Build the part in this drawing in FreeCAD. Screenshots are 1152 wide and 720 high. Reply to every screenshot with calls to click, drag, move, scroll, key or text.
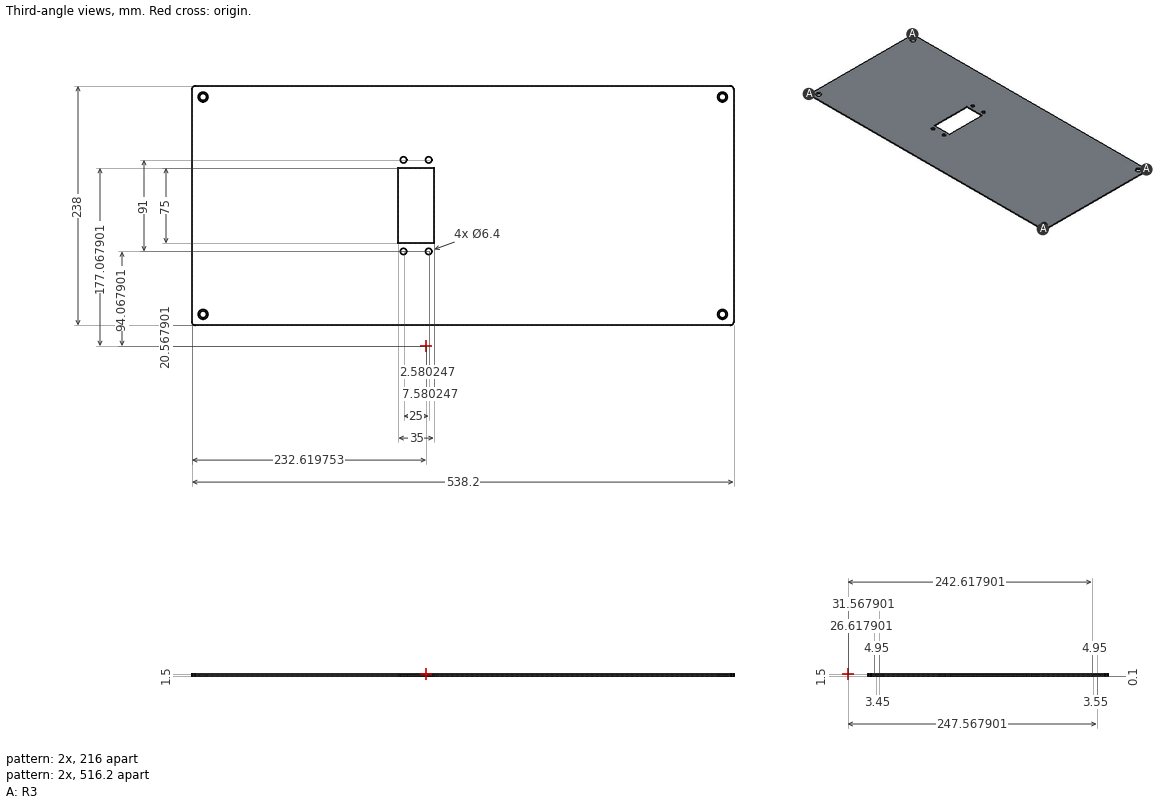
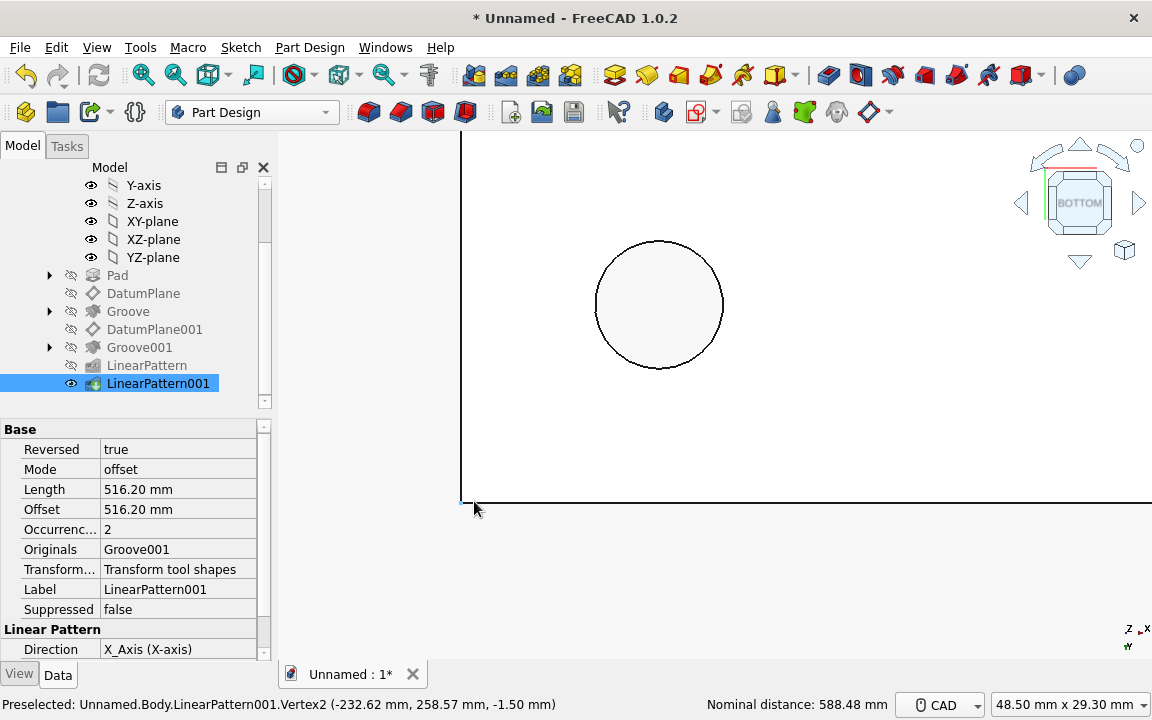
click(144, 76)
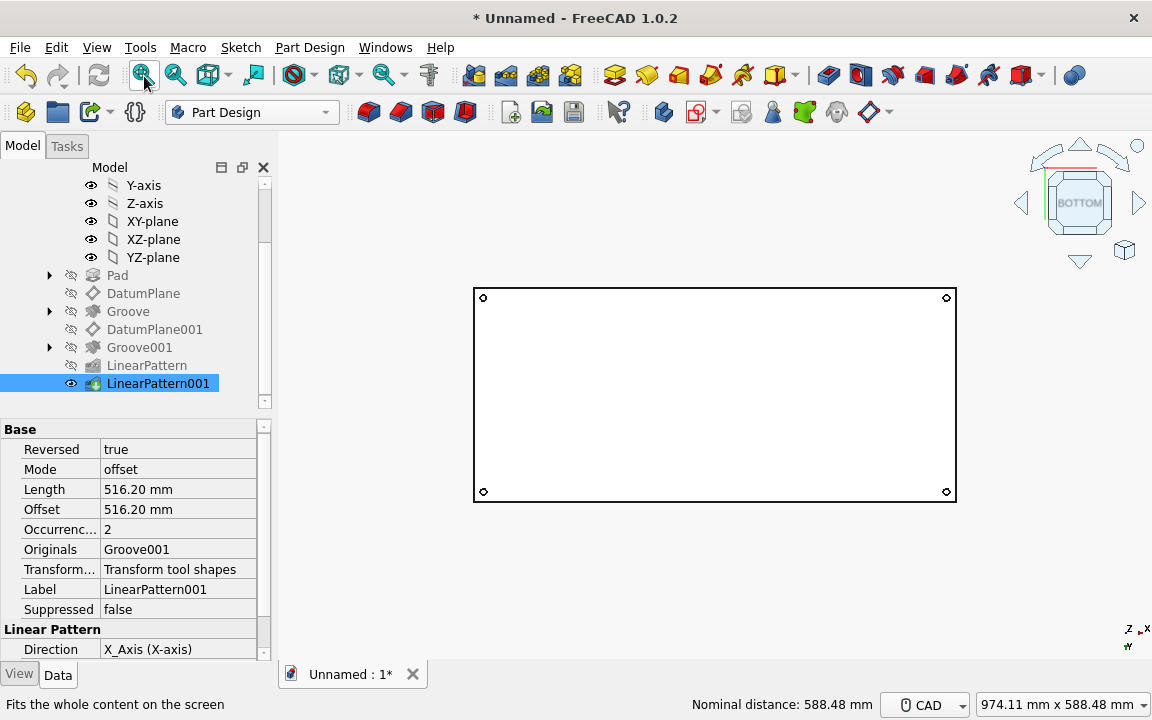
key(4)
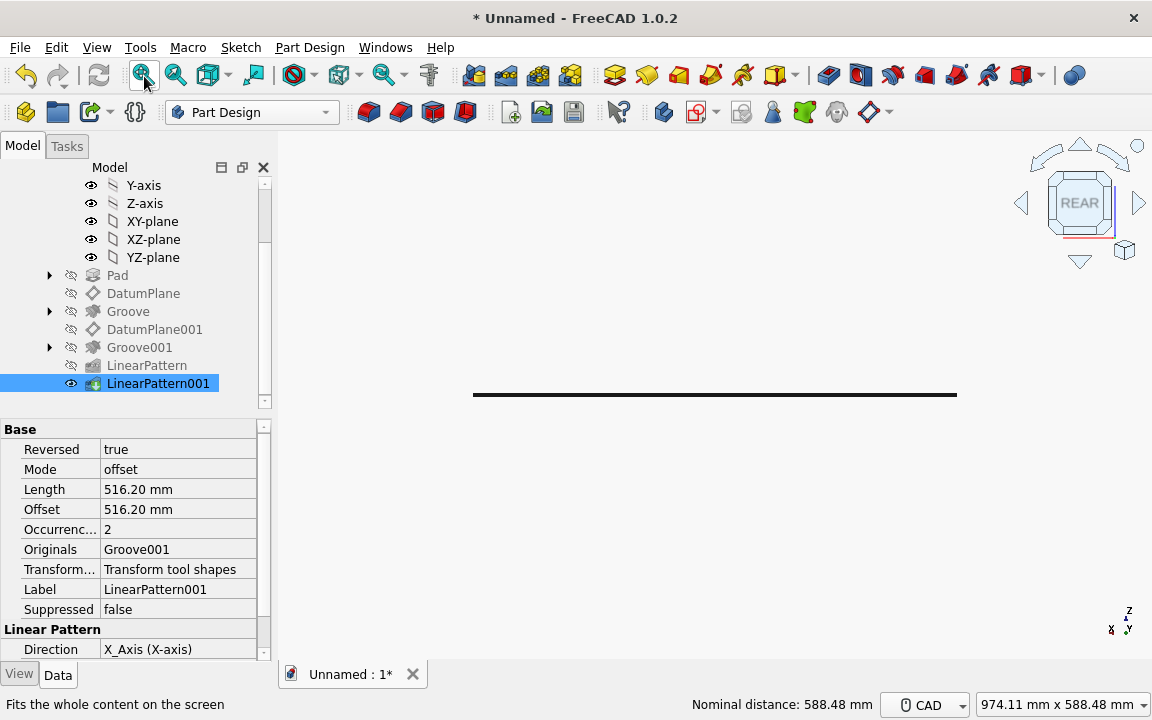
scroll(956, 394, up, 15)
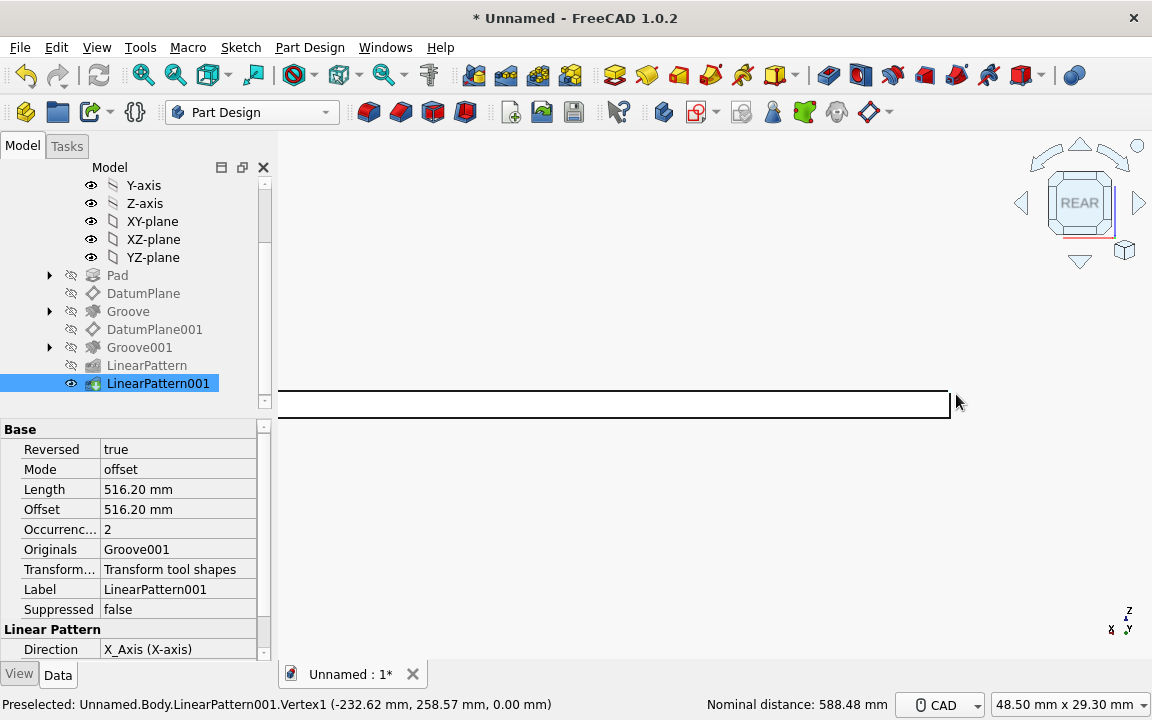
click(950, 404, ctrl)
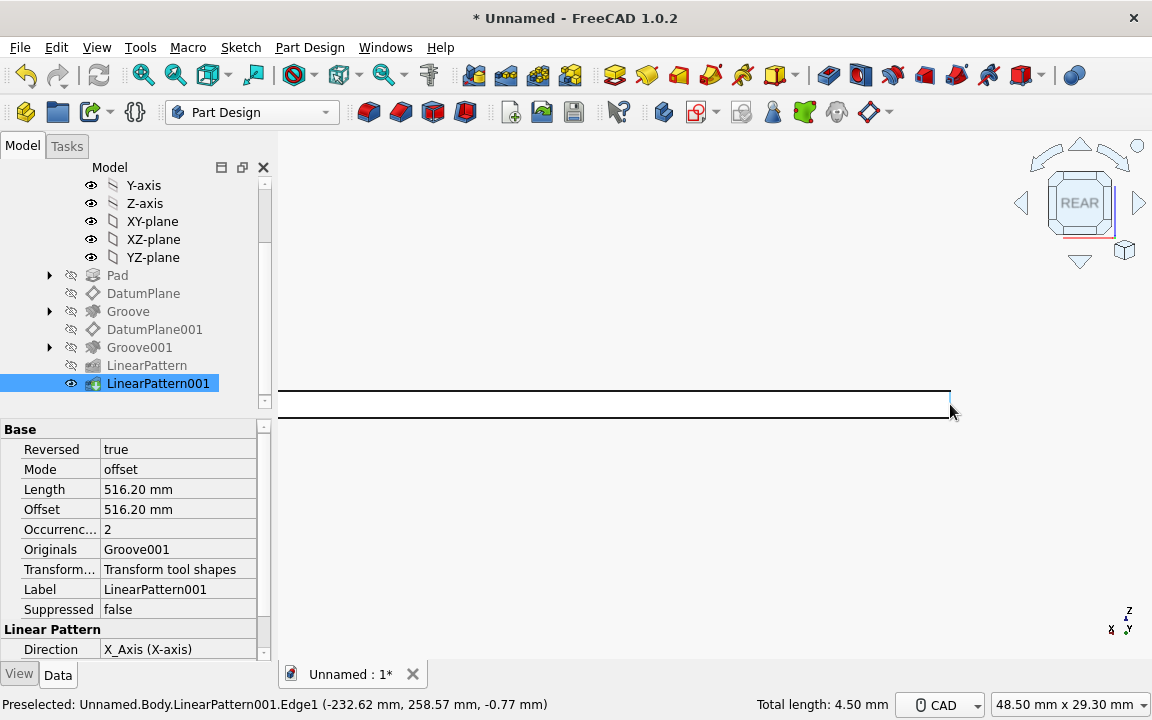
click(144, 76)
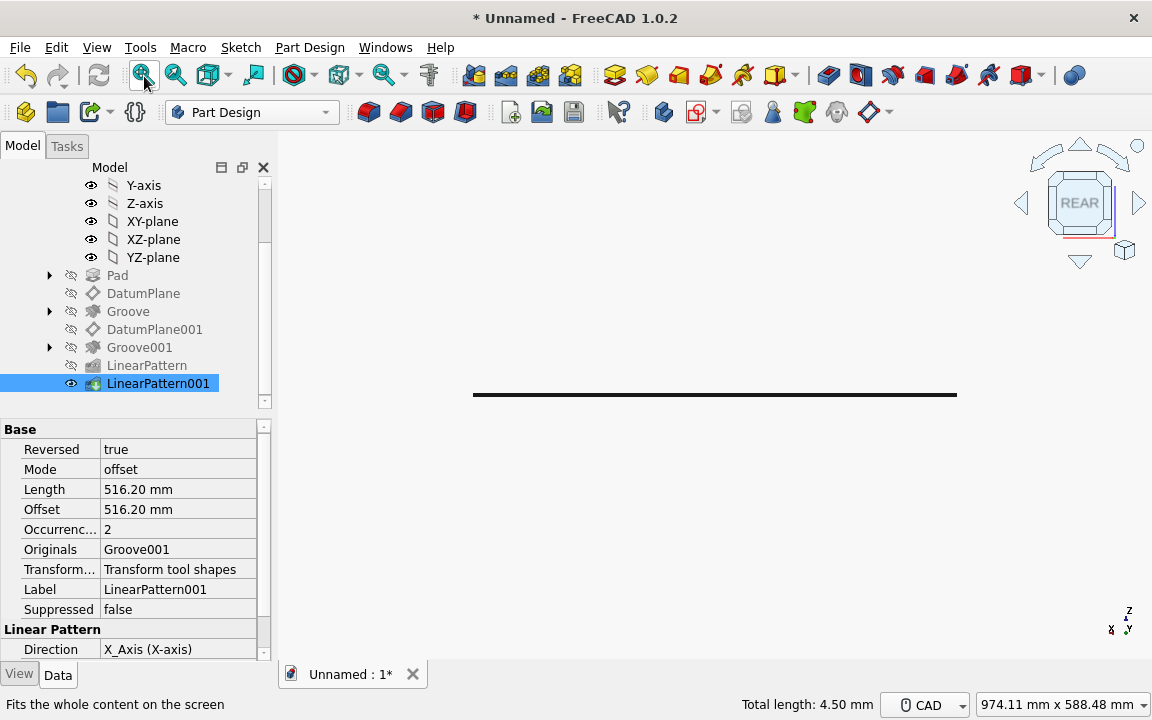
key(6)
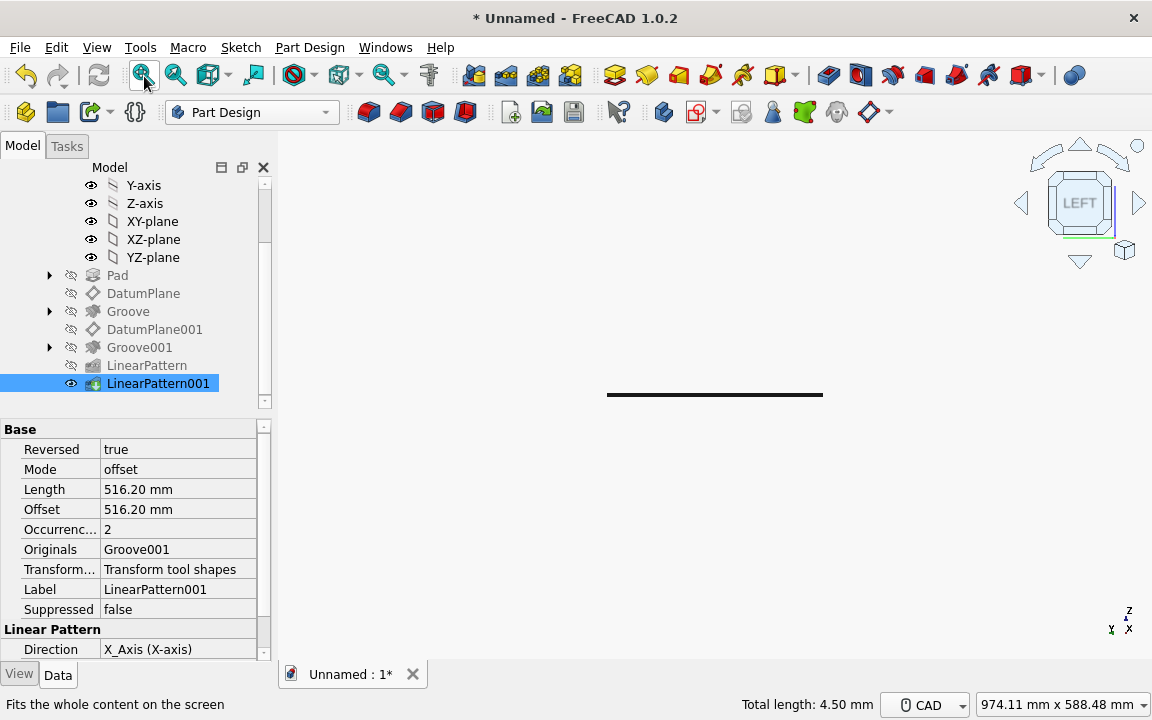
click(144, 76)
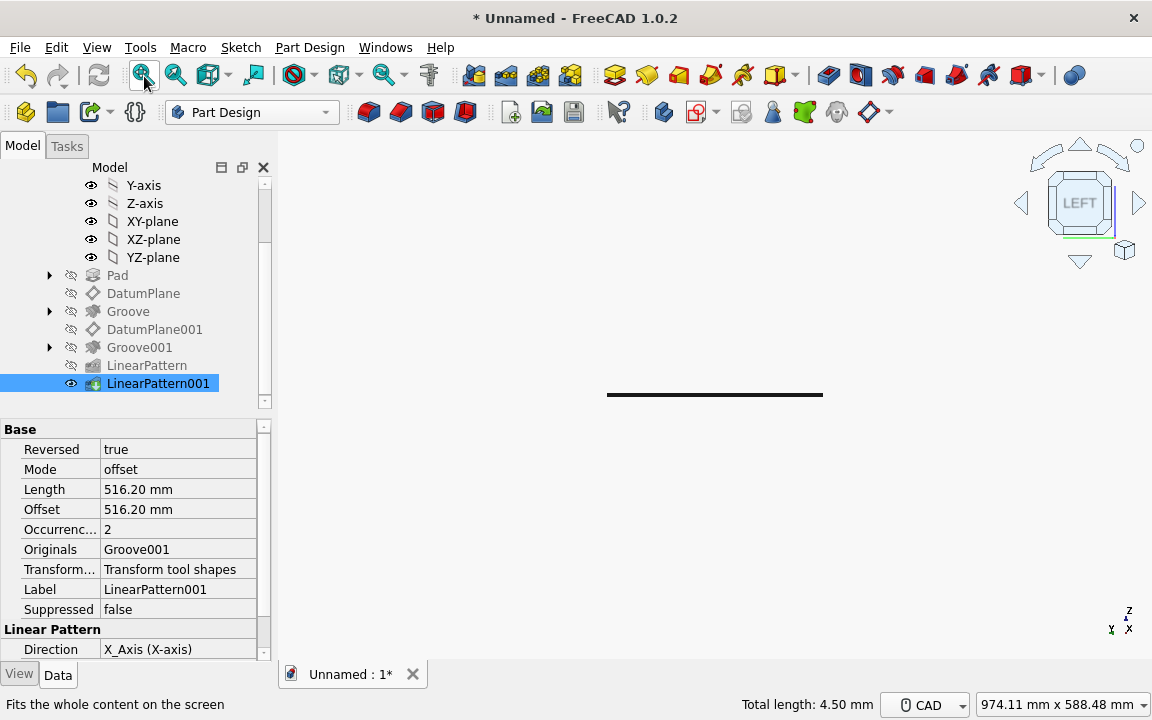
scroll(822, 394, up, 15)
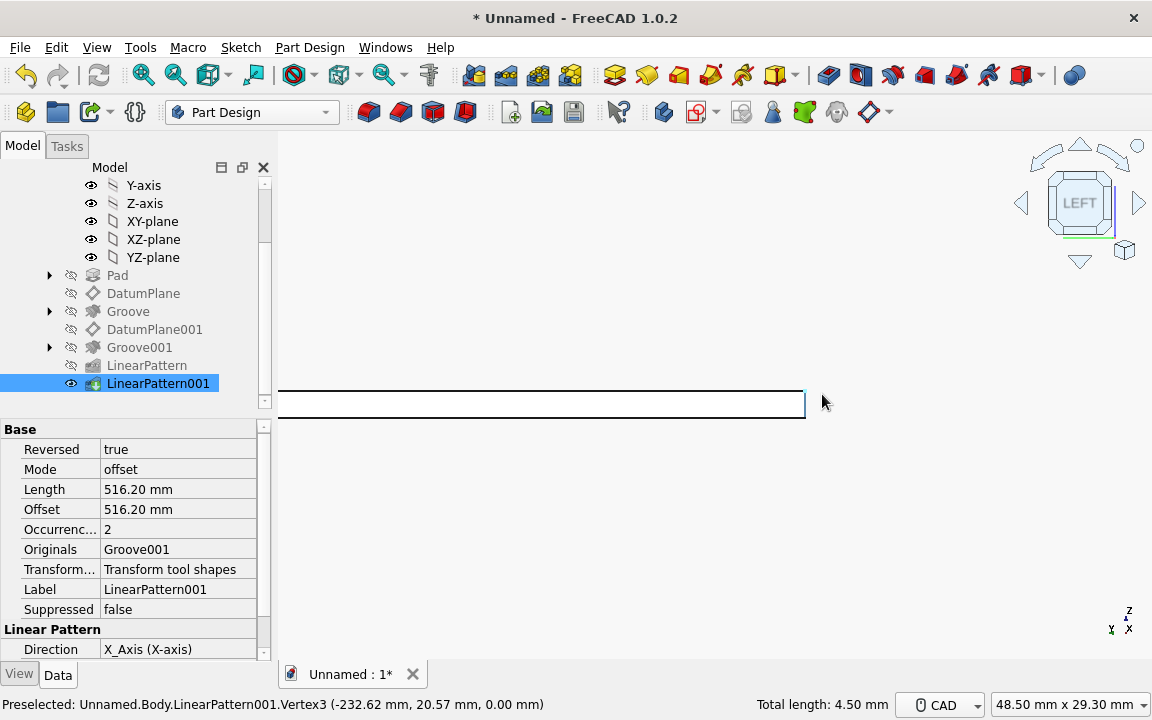
click(144, 76)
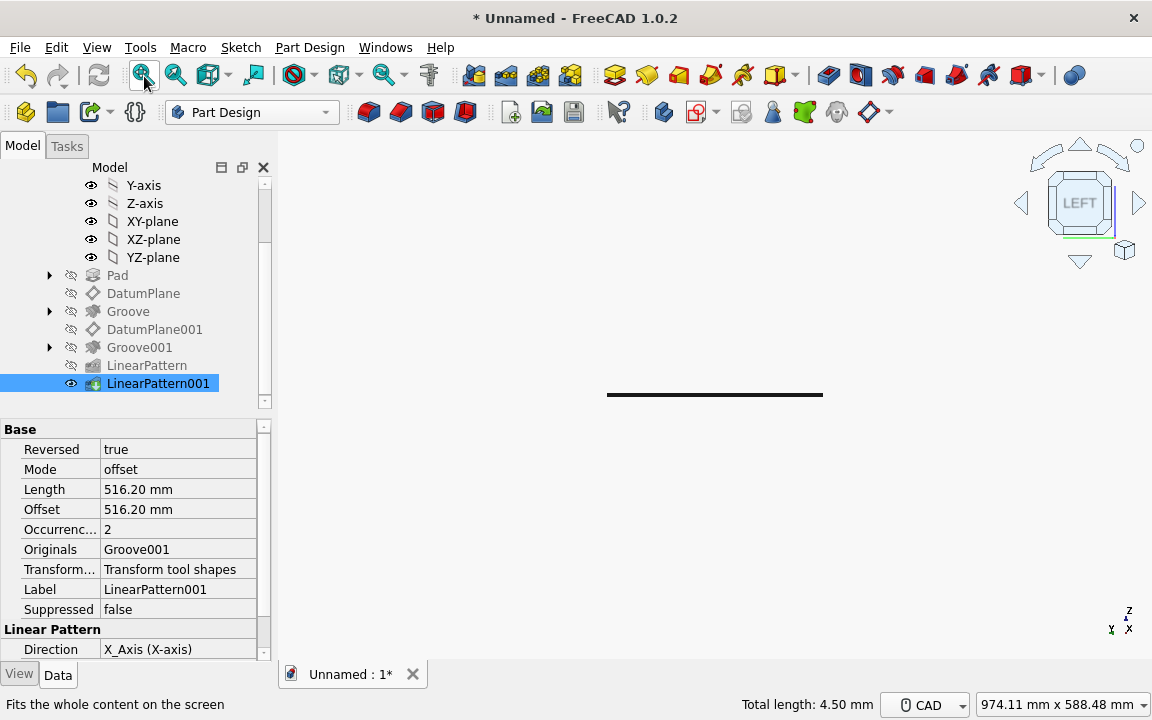
key(v)
key(3)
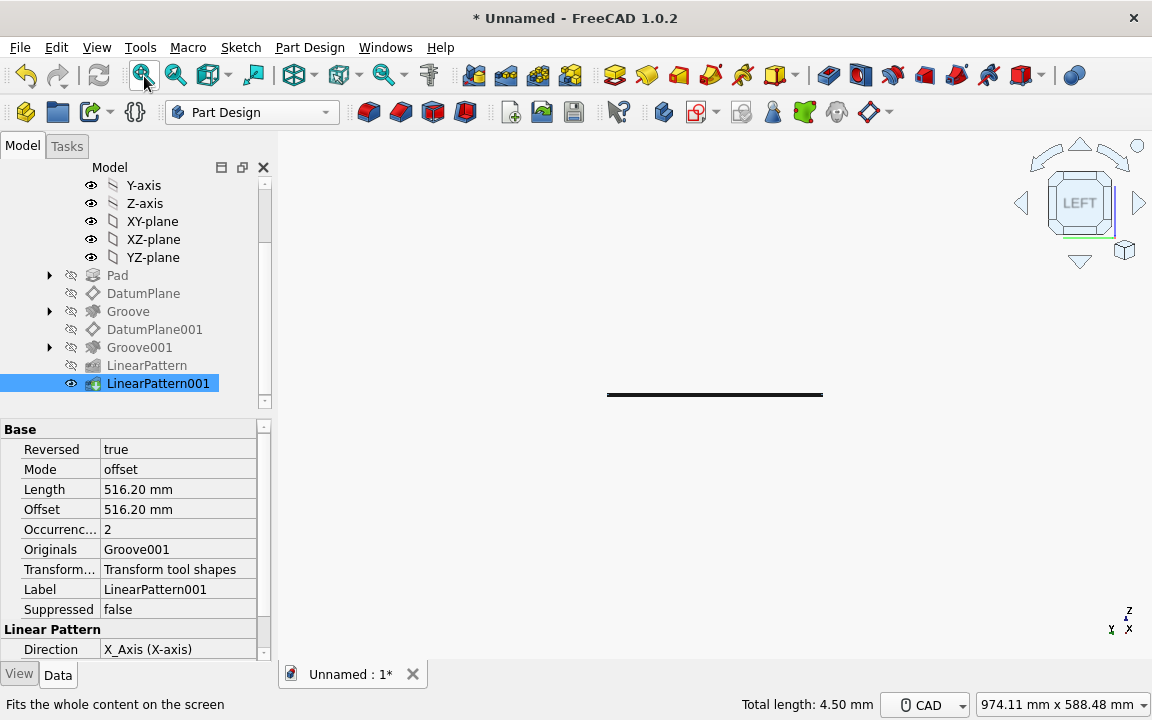
key(0)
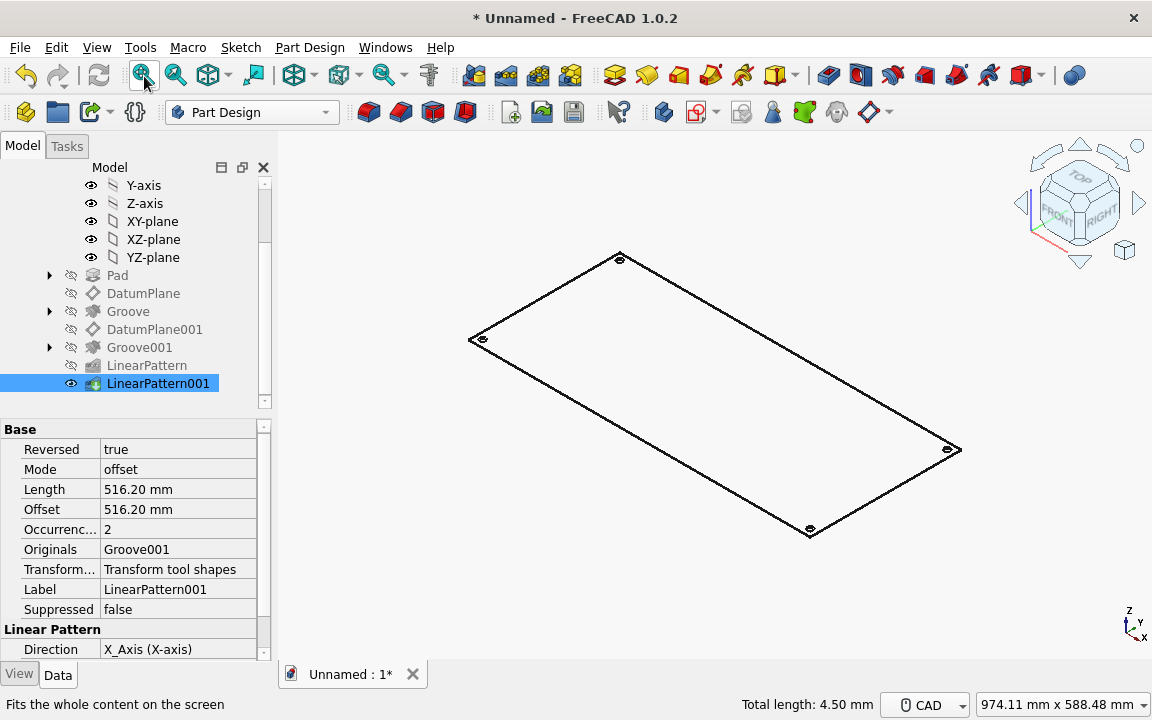
scroll(810, 536, up, 15)